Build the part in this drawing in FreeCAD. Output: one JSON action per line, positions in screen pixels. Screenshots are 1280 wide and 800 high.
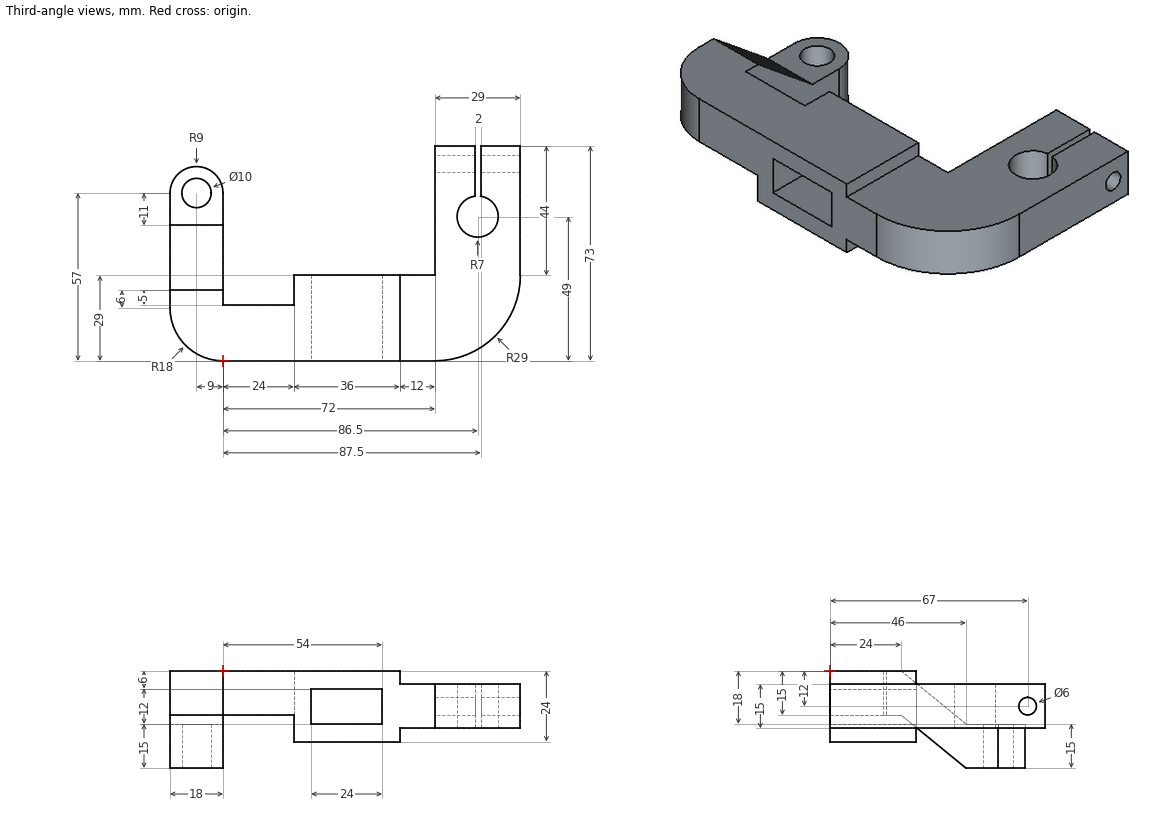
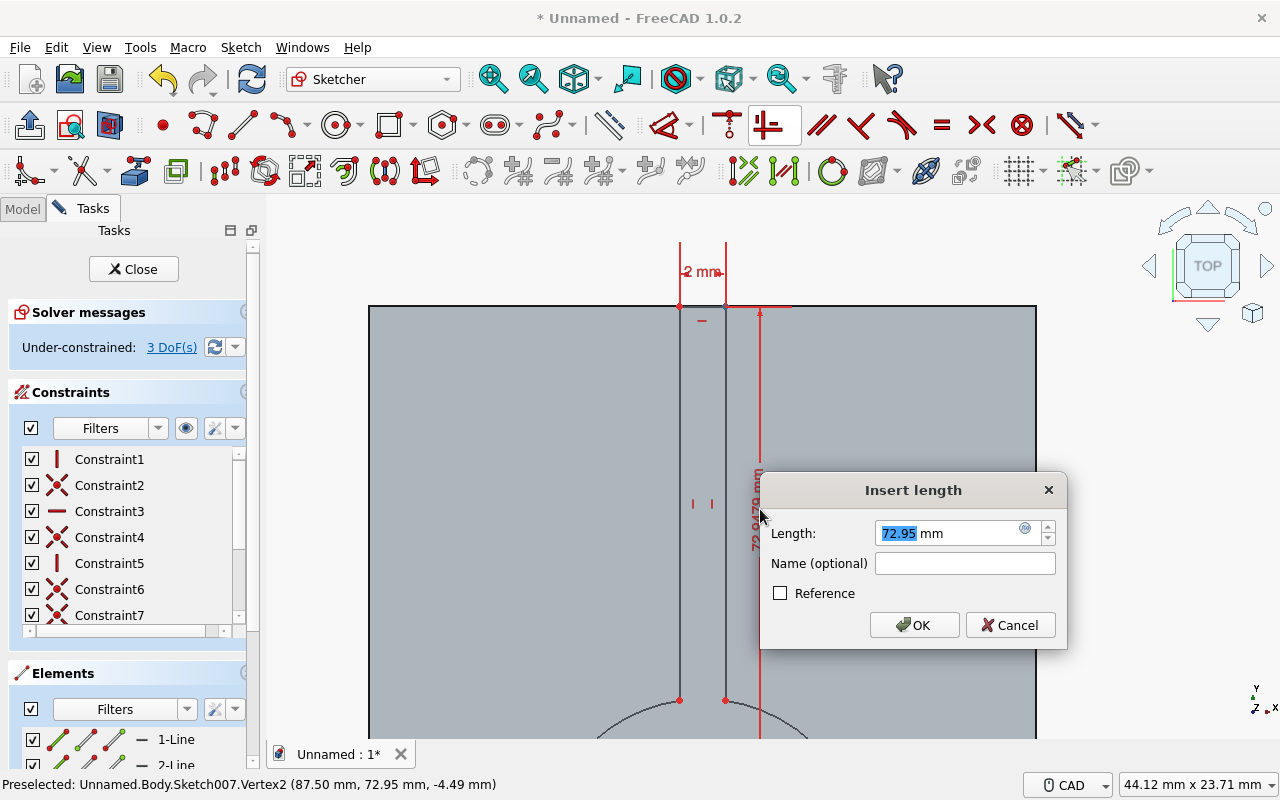
{"action": "type", "text": "73"}
{"action": "key", "text": "Return"}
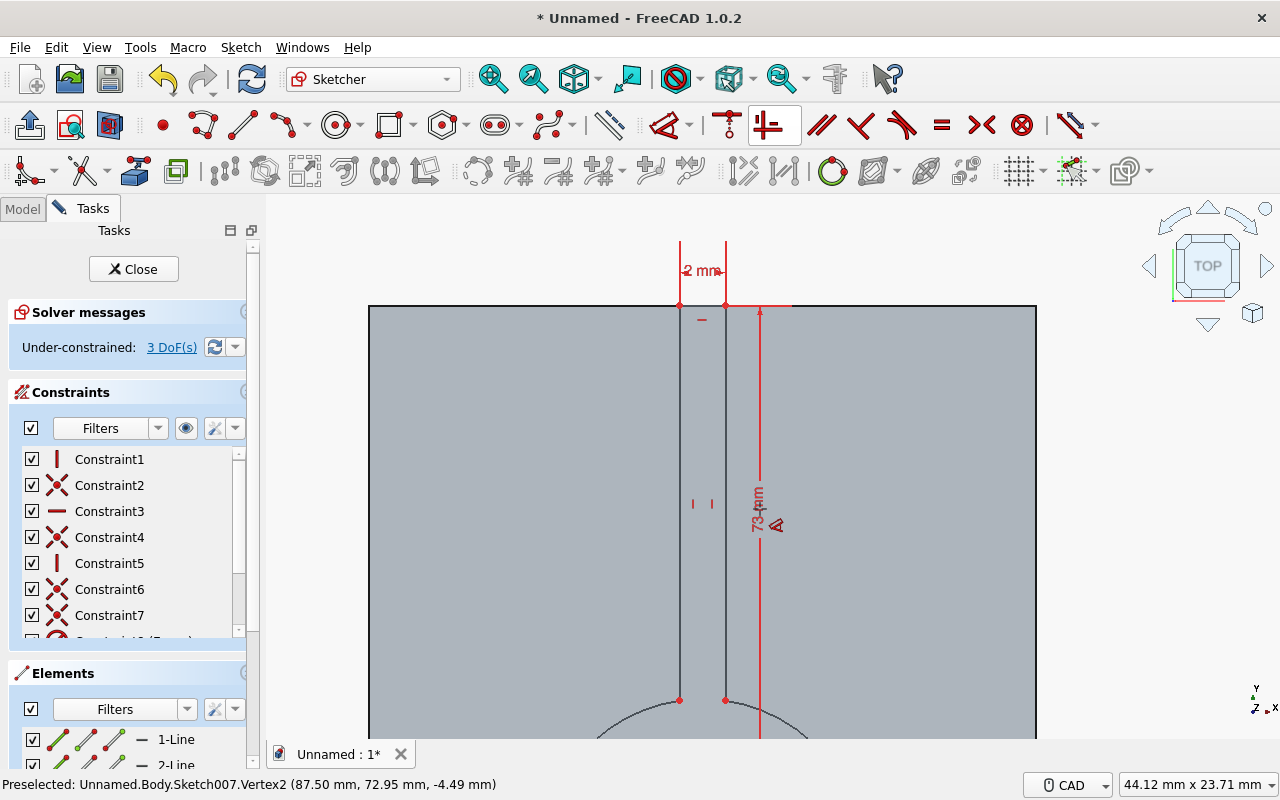
{"action": "scroll", "coordinate": [706, 307], "scroll_direction": "down", "scroll_amount": 4}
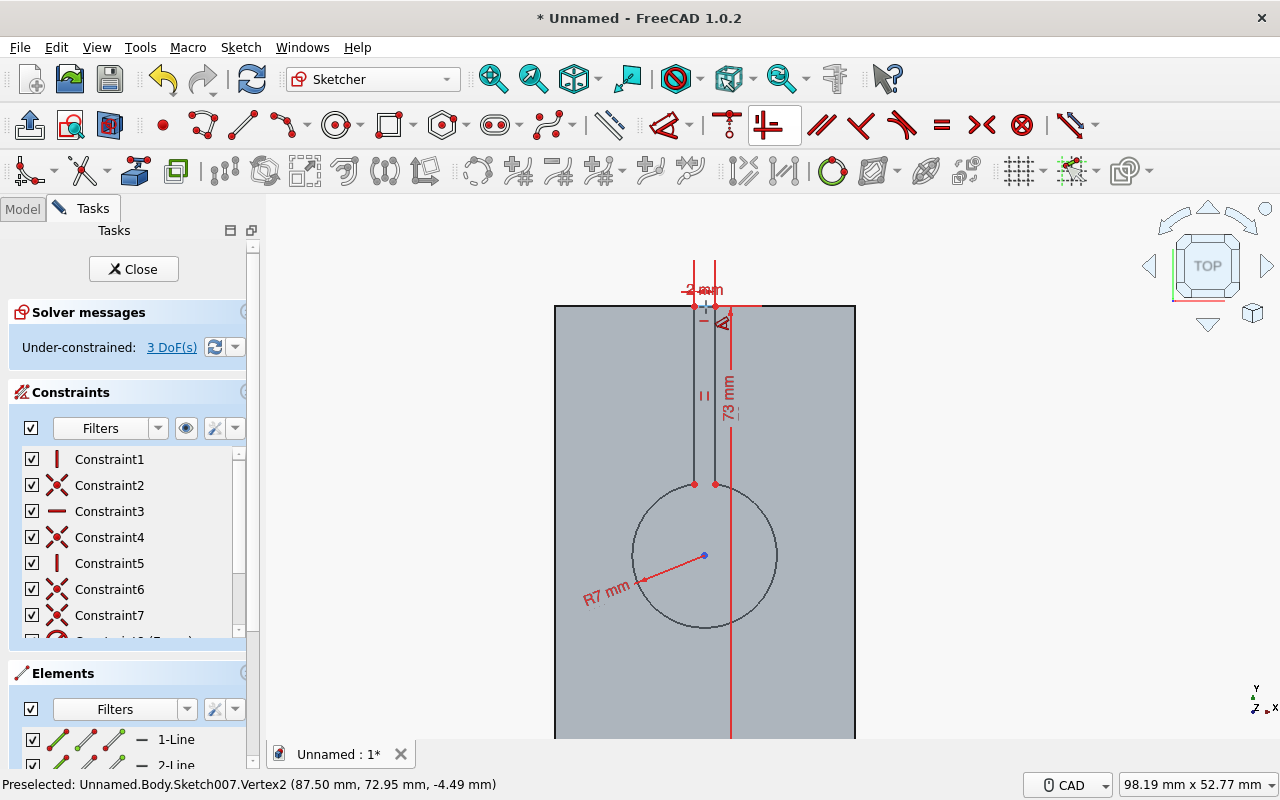
{"action": "left_click", "coordinate": [705, 556]}
{"action": "left_click", "coordinate": [739, 598]}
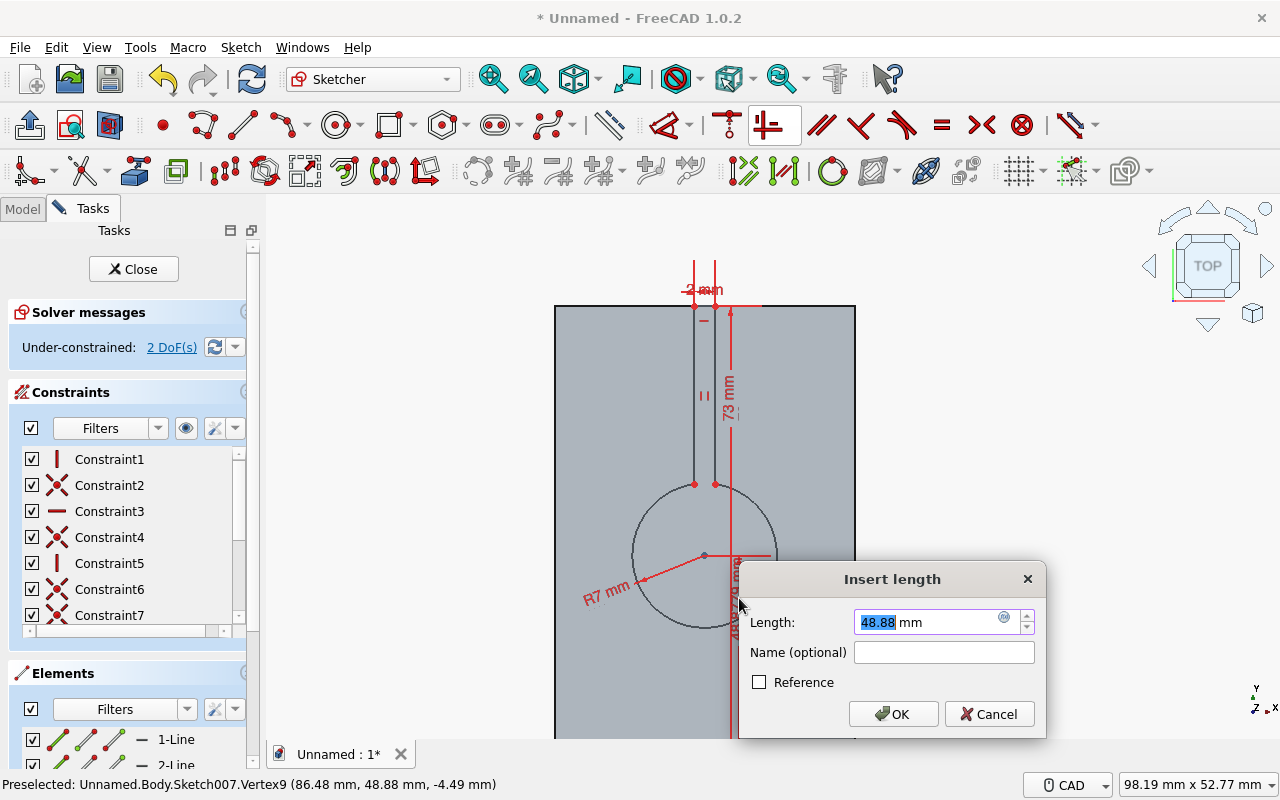
{"action": "type", "text": "49"}
{"action": "key", "text": "Return"}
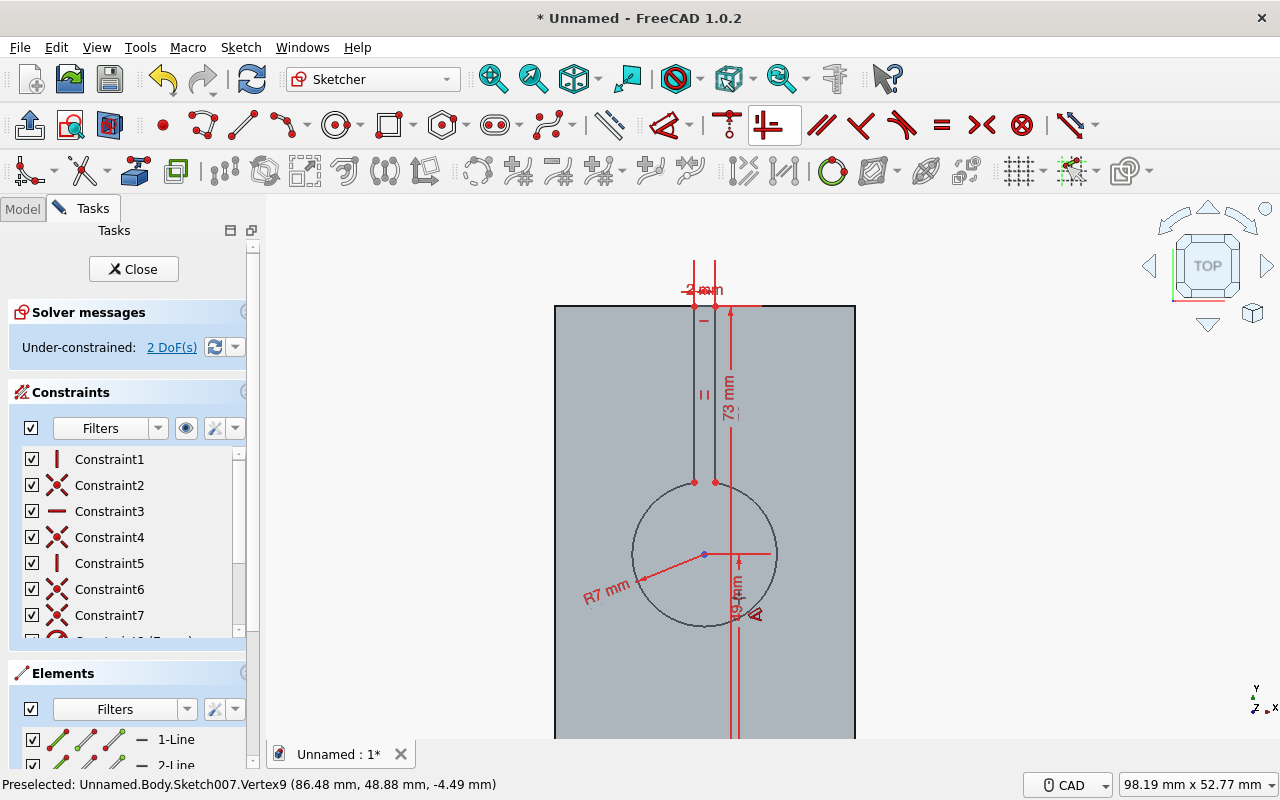
{"action": "left_click", "coordinate": [715, 483]}
{"action": "left_click", "coordinate": [505, 449]}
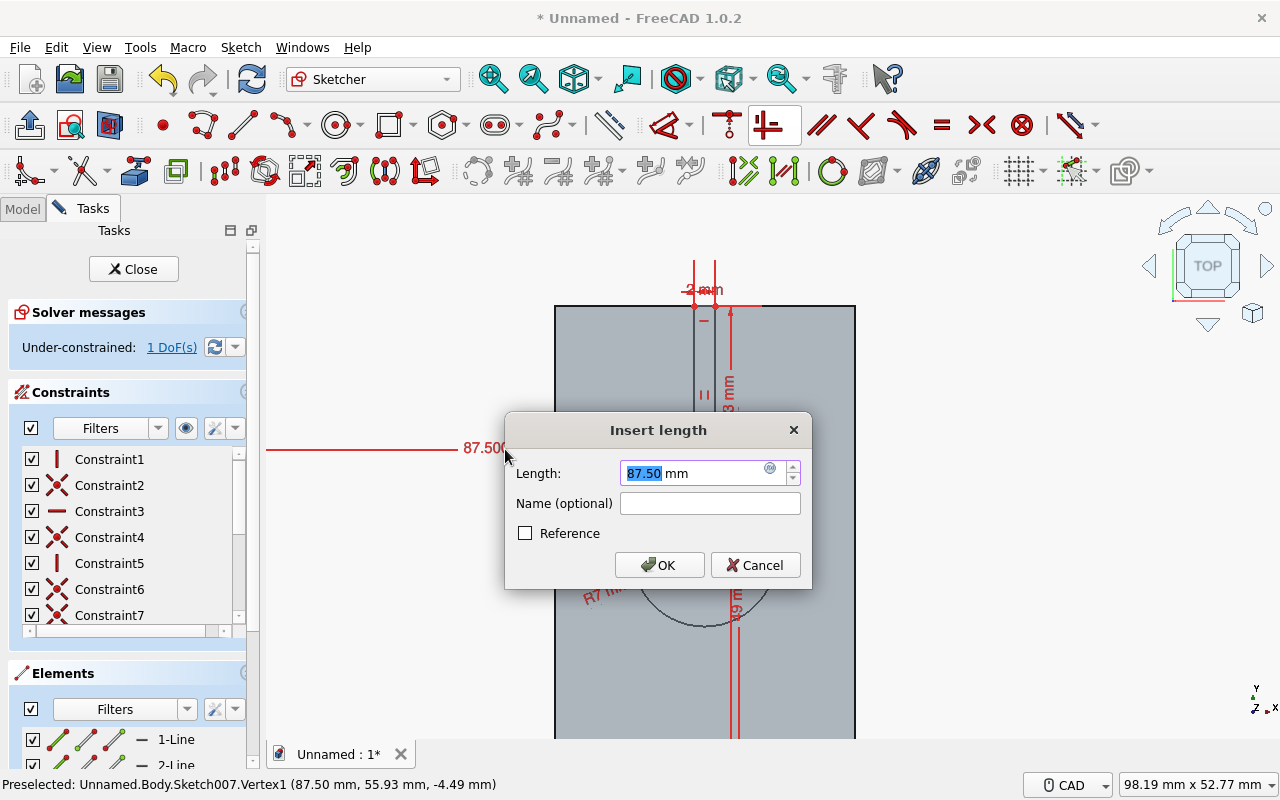
{"action": "type", "text": "87.5"}
{"action": "key", "text": "Return"}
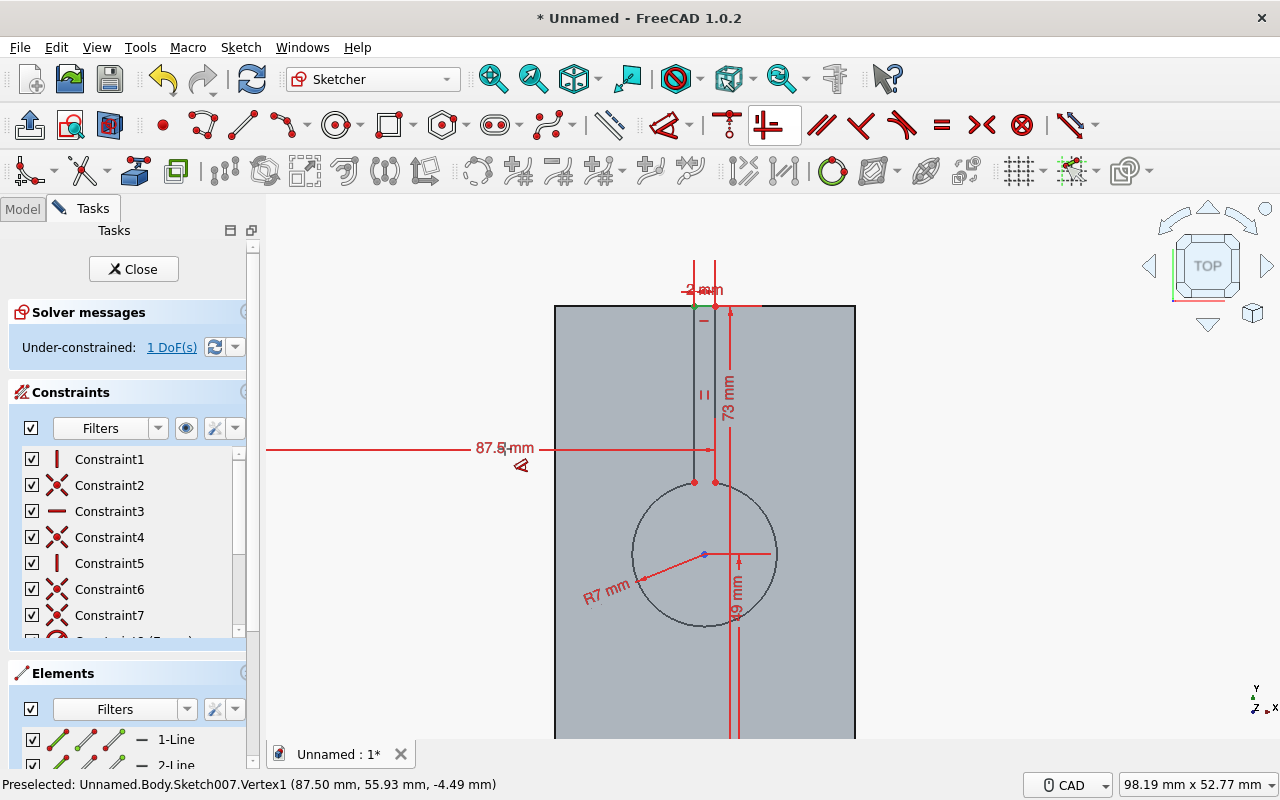
{"action": "left_click", "coordinate": [705, 554]}
{"action": "left_click", "coordinate": [499, 520]}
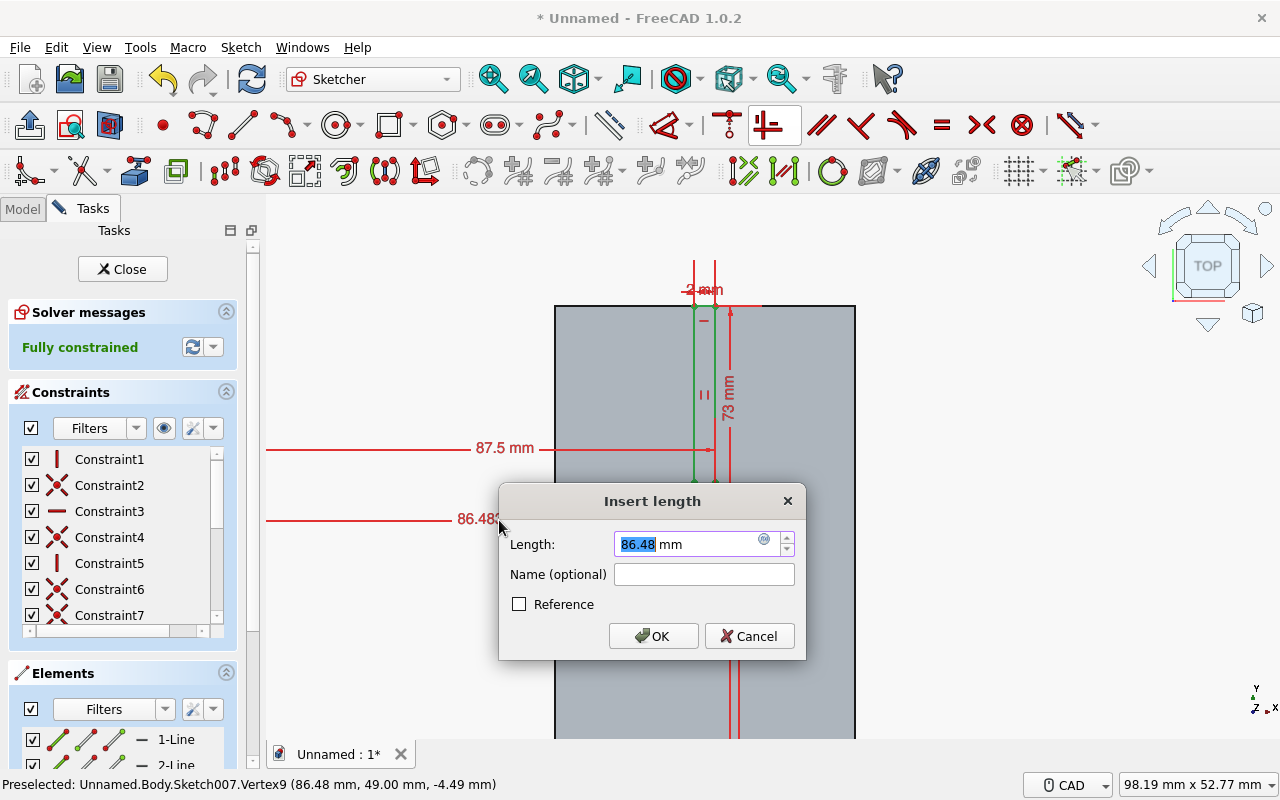
{"action": "type", "text": "86.5"}
{"action": "key", "text": "Return"}
{"action": "key", "text": "Escape"}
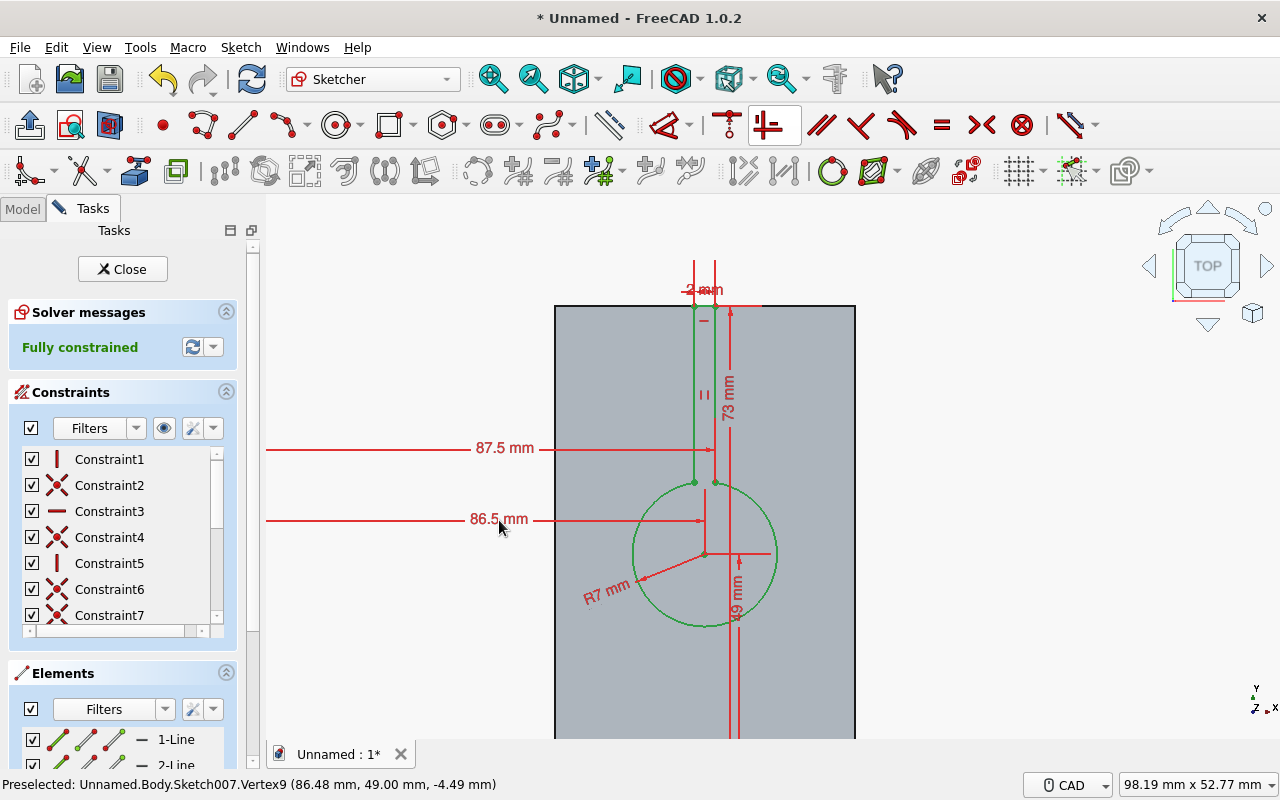
{"action": "left_click", "coordinate": [123, 269]}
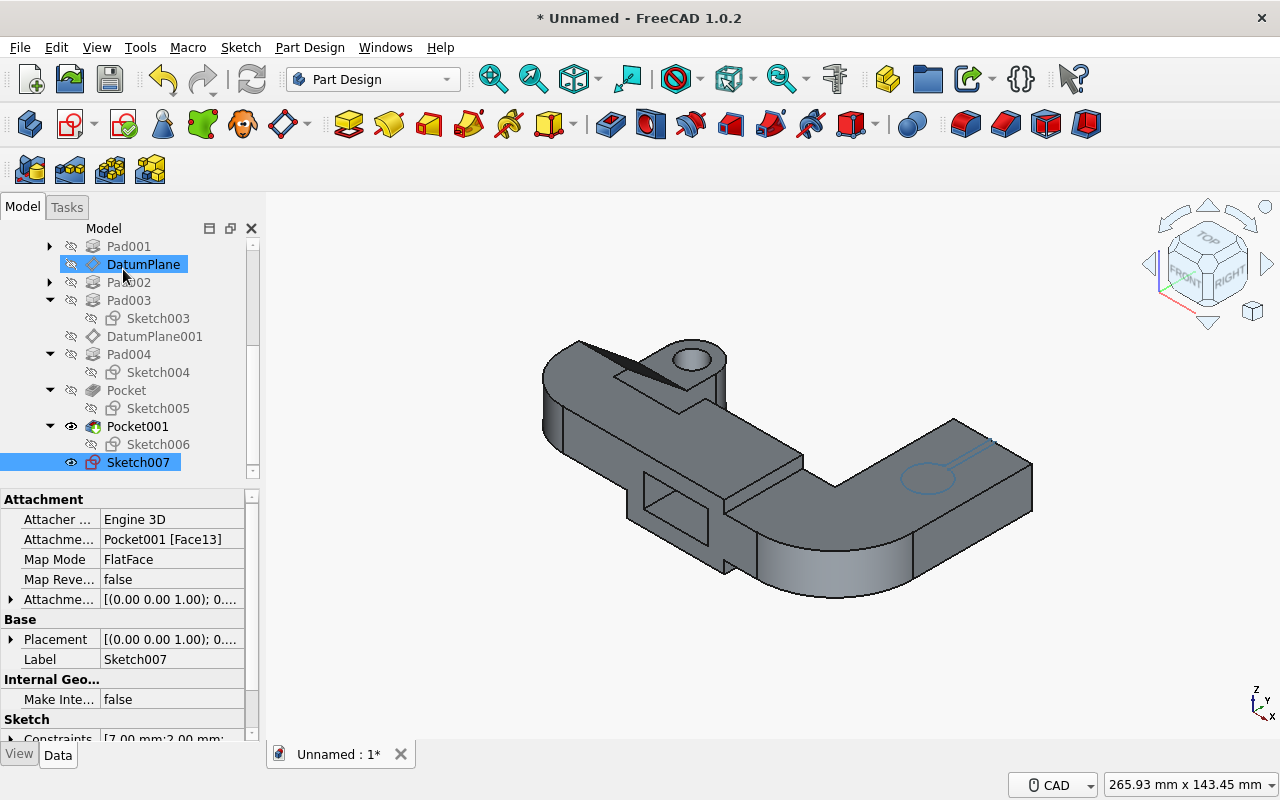
{"action": "left_click", "coordinate": [612, 124]}